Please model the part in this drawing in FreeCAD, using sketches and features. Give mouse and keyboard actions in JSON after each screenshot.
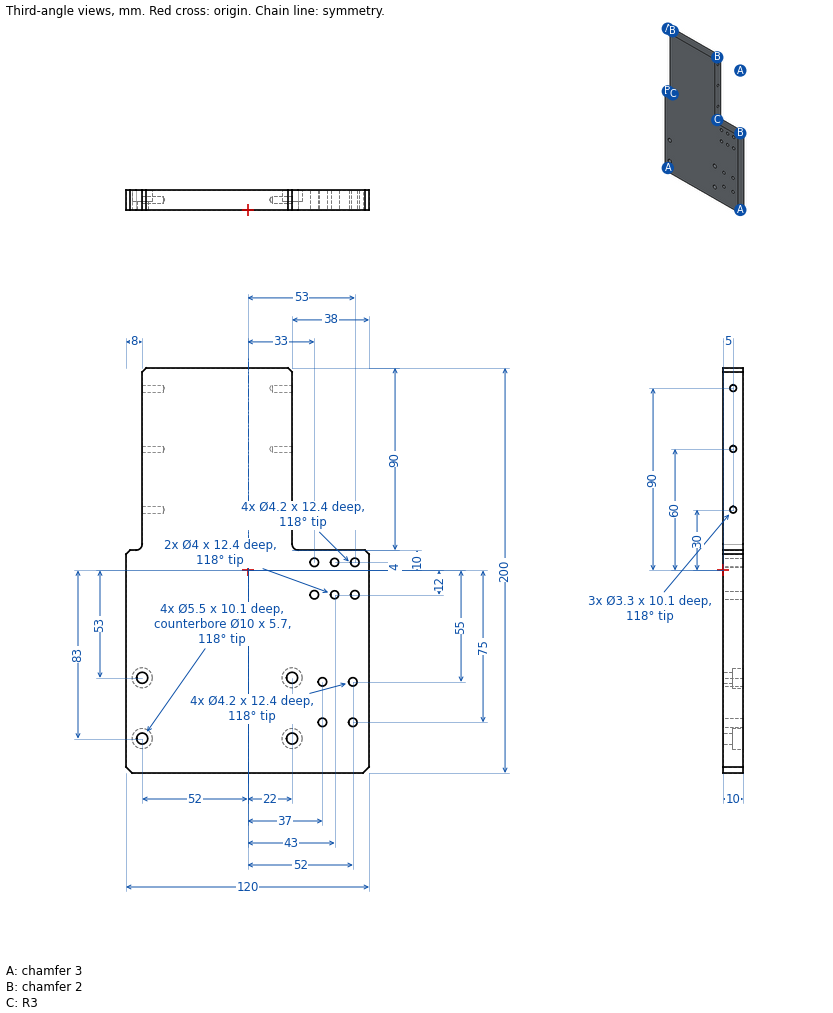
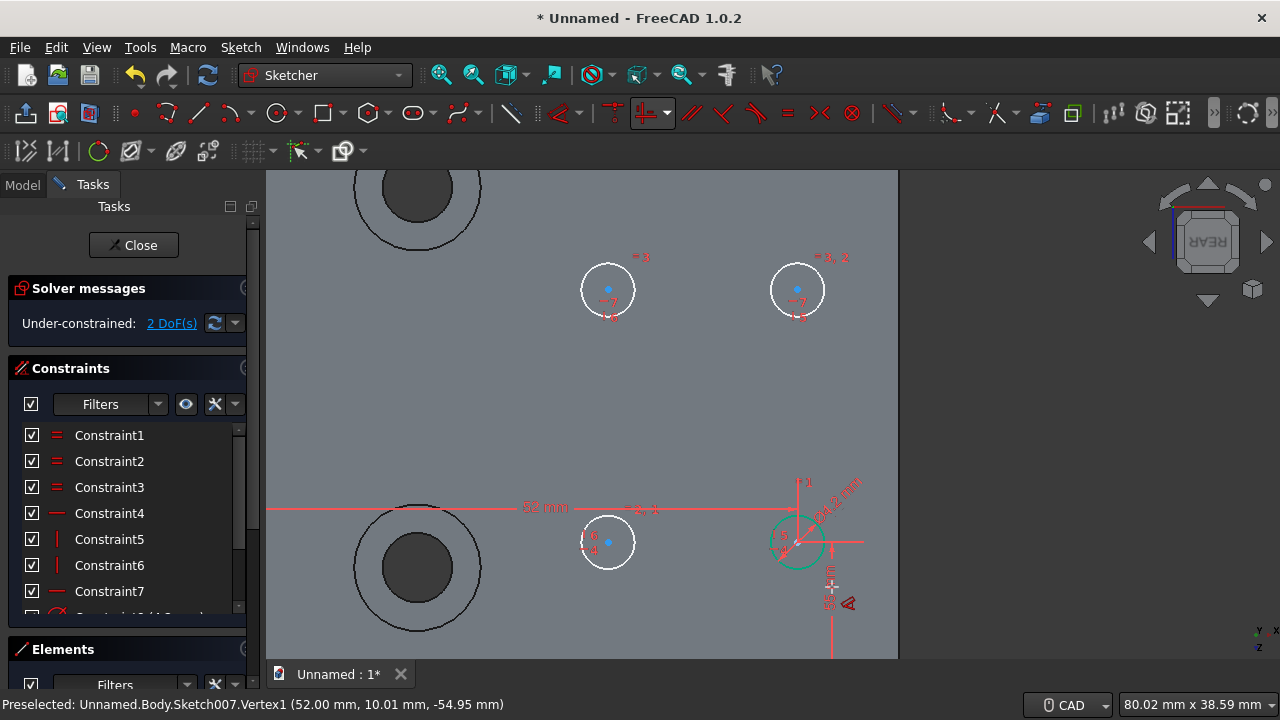
{"action": "left_click", "coordinate": [608, 542]}
{"action": "left_click", "coordinate": [451, 508]}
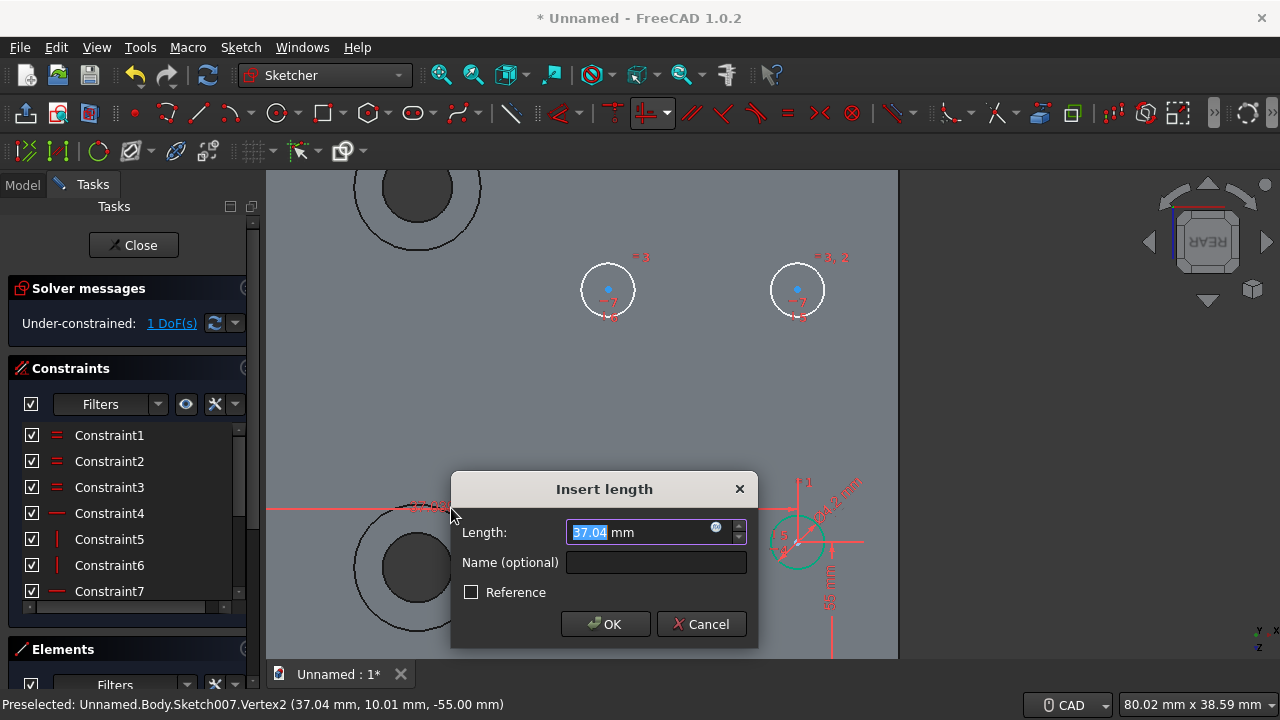
{"action": "type", "text": "37"}
{"action": "key", "text": "Return"}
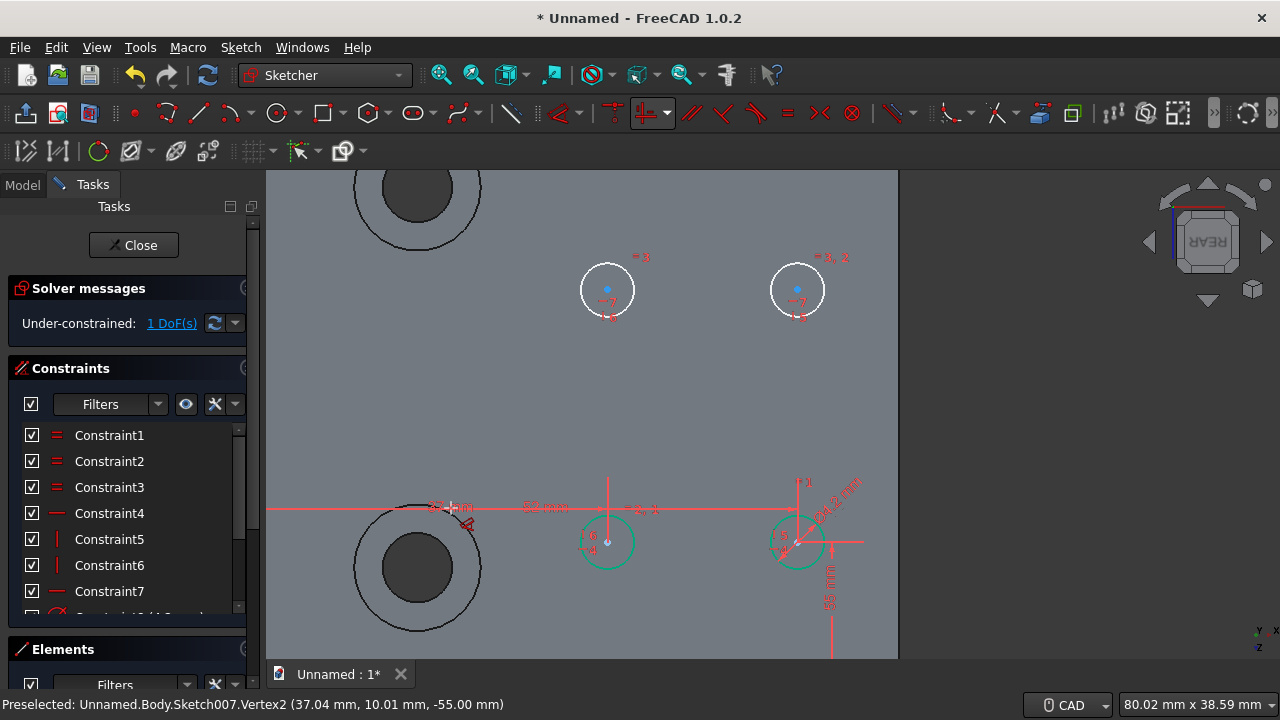
{"action": "left_click", "coordinate": [798, 290]}
{"action": "left_click", "coordinate": [832, 461]}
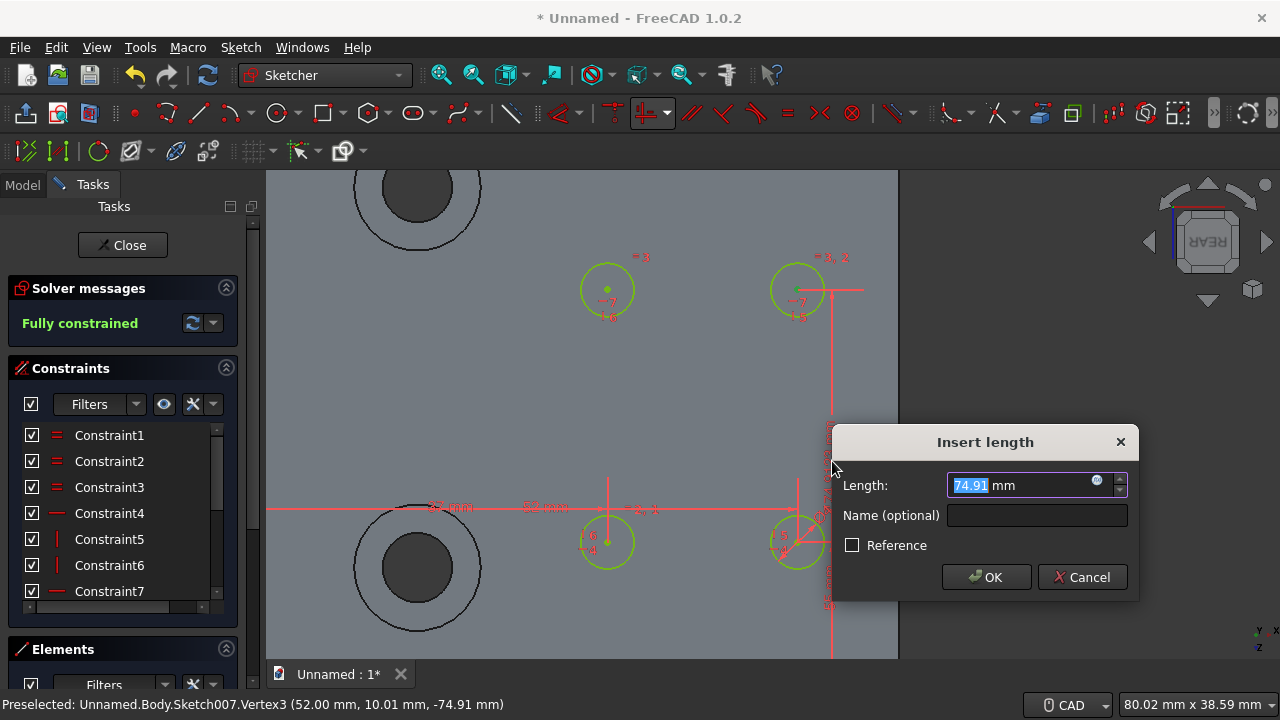
{"action": "type", "text": "75"}
{"action": "key", "text": "Return"}
{"action": "key", "text": "Escape"}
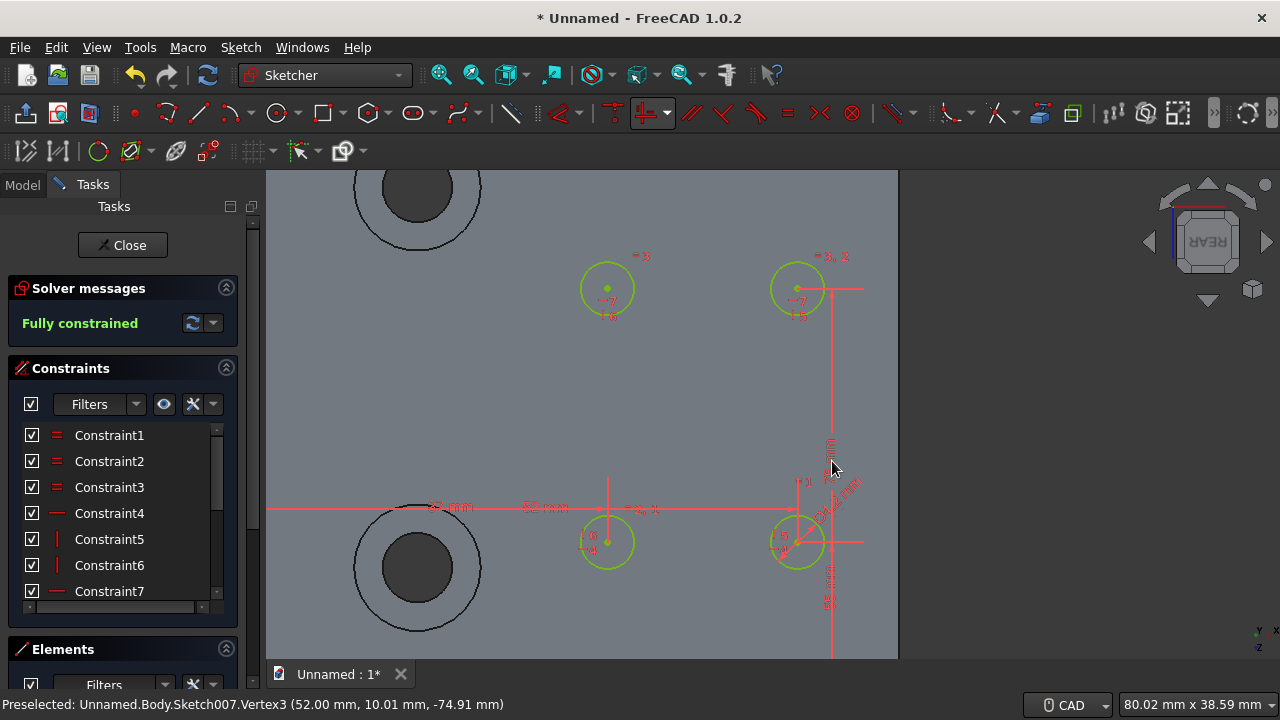
{"action": "left_click", "coordinate": [123, 245]}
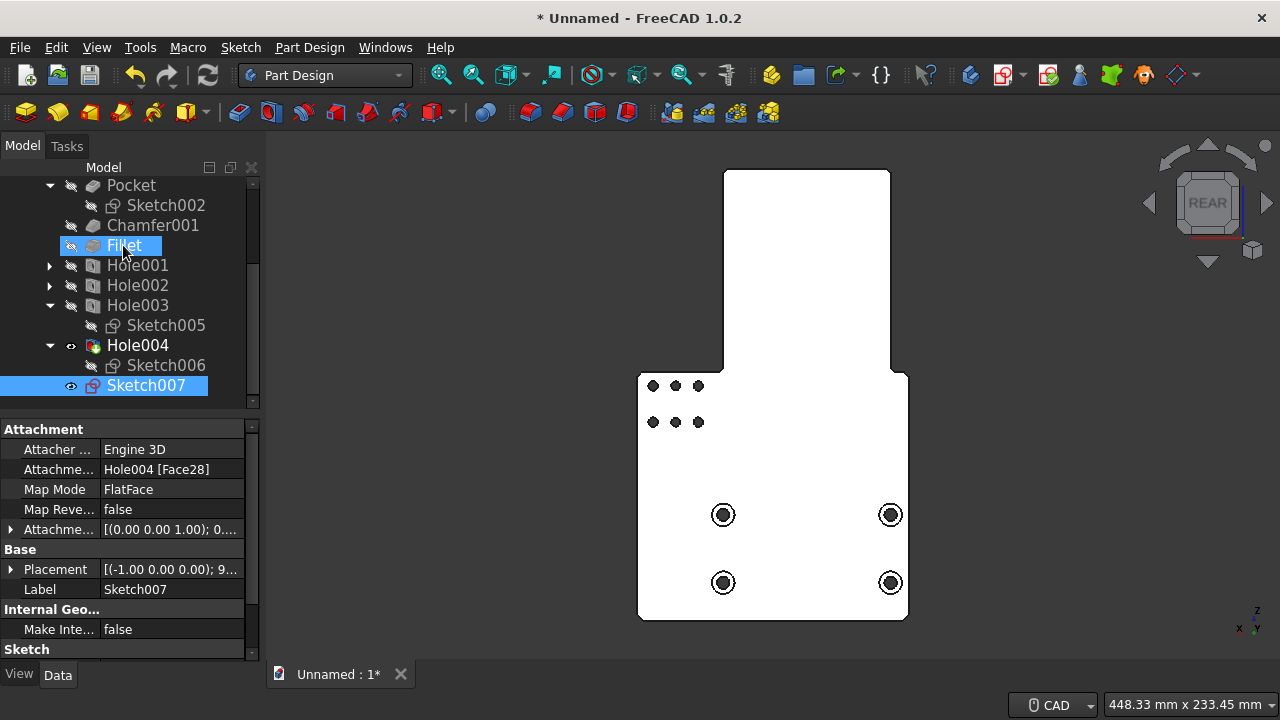
{"action": "left_click", "coordinate": [272, 112]}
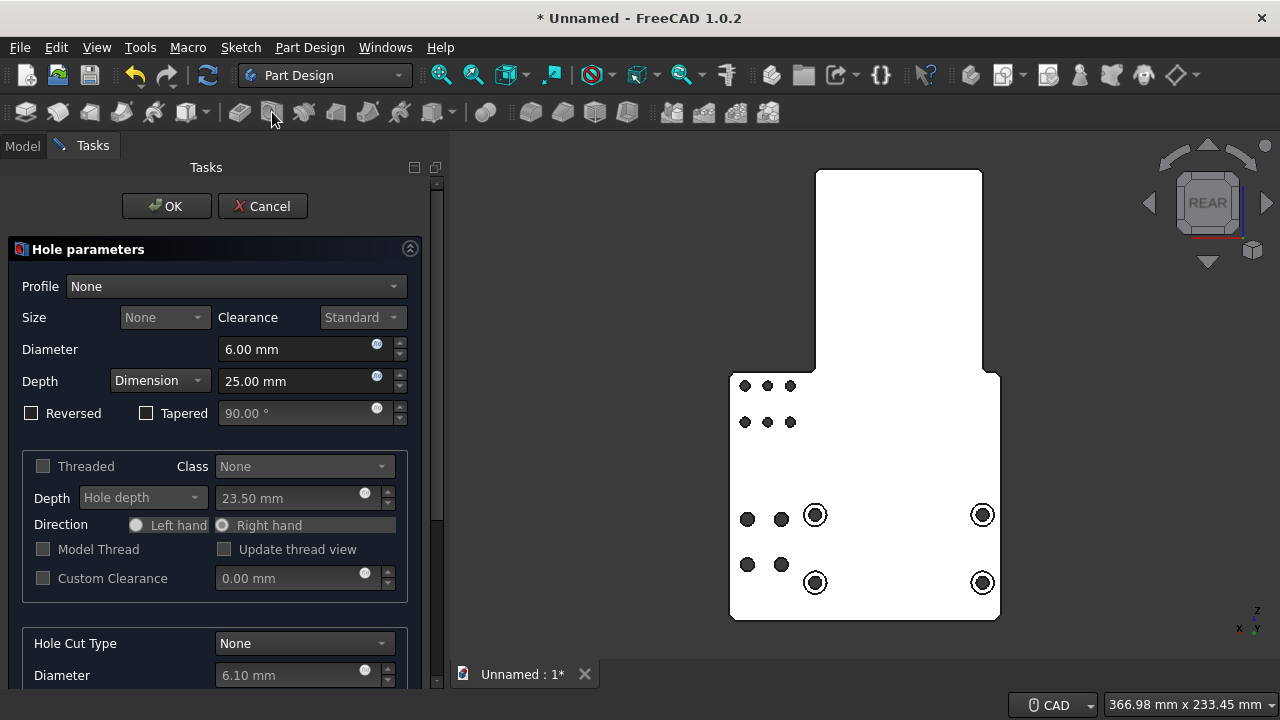
{"action": "triple_click", "coordinate": [305, 349]}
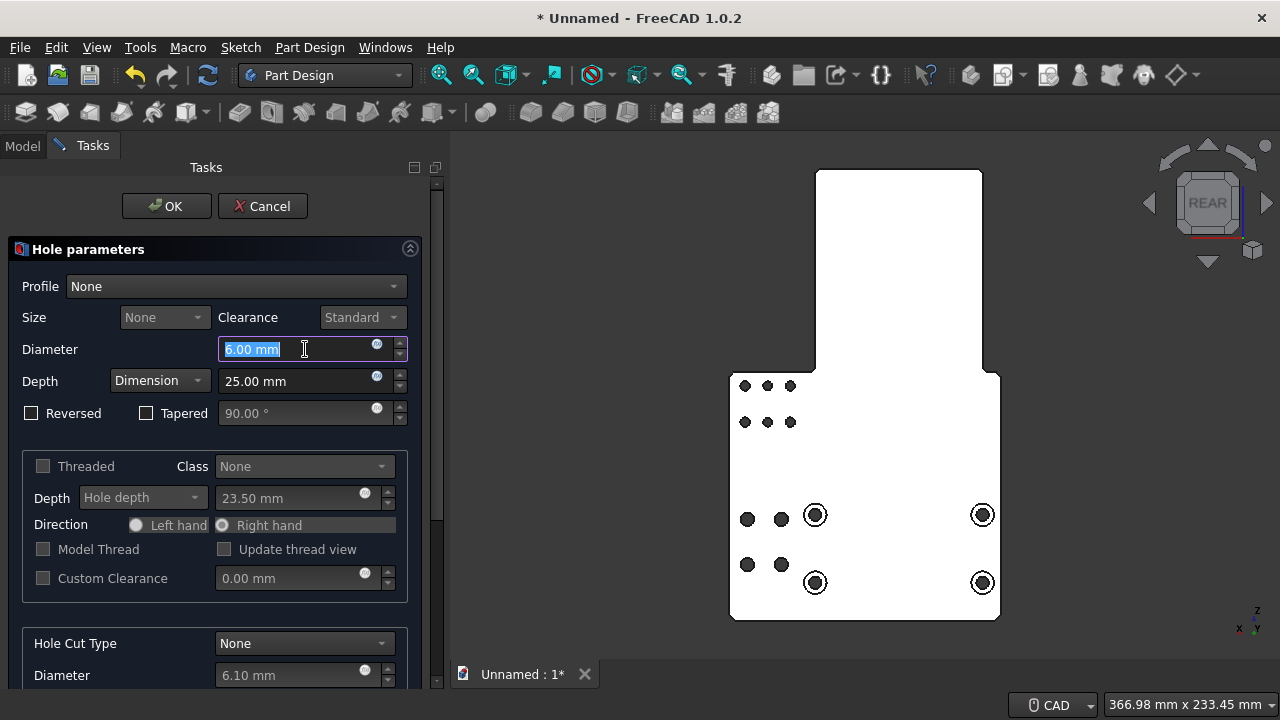
{"action": "type", "text": "4.2"}
{"action": "key", "text": "Tab"}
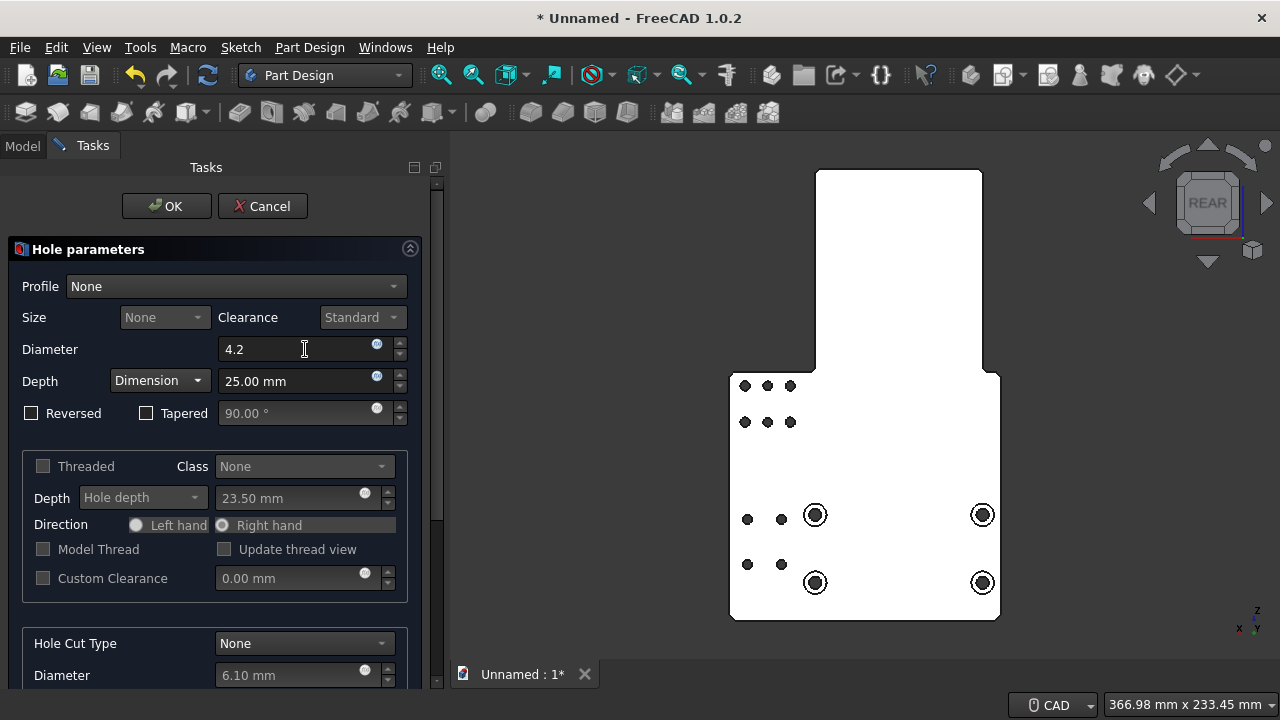
{"action": "triple_click", "coordinate": [305, 381]}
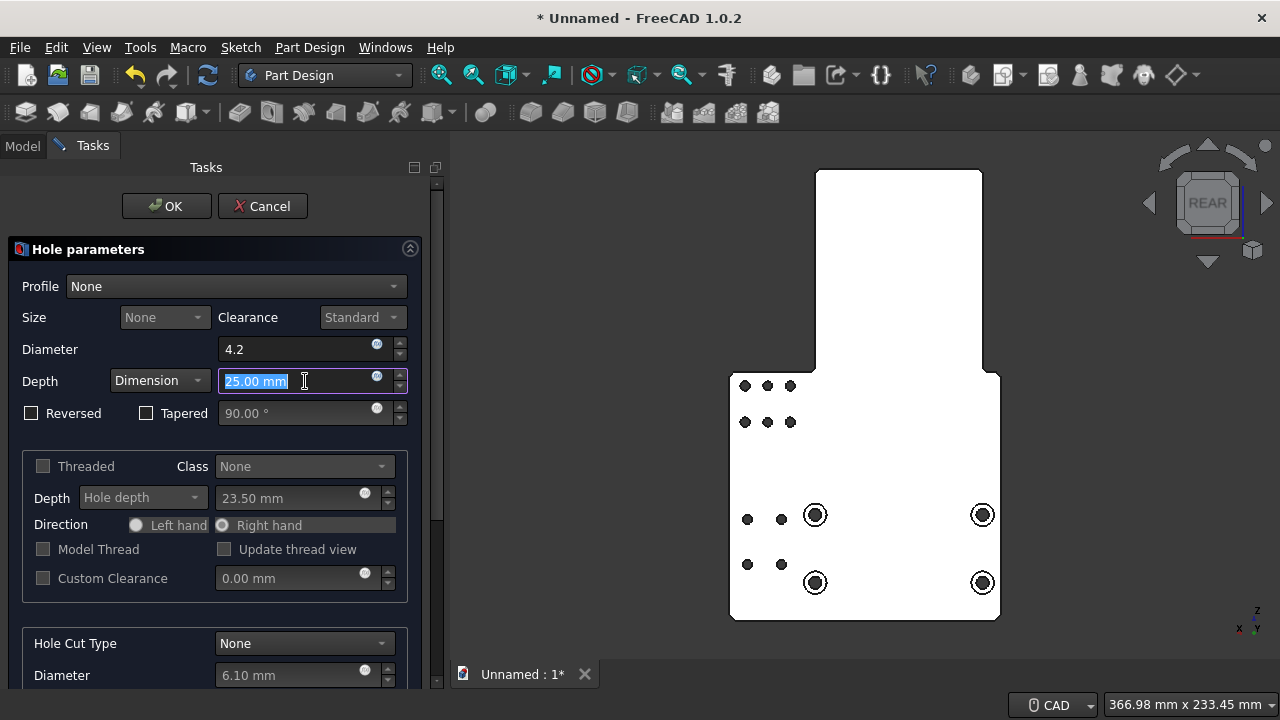
{"action": "type", "text": "12.4"}
{"action": "key", "text": "Tab"}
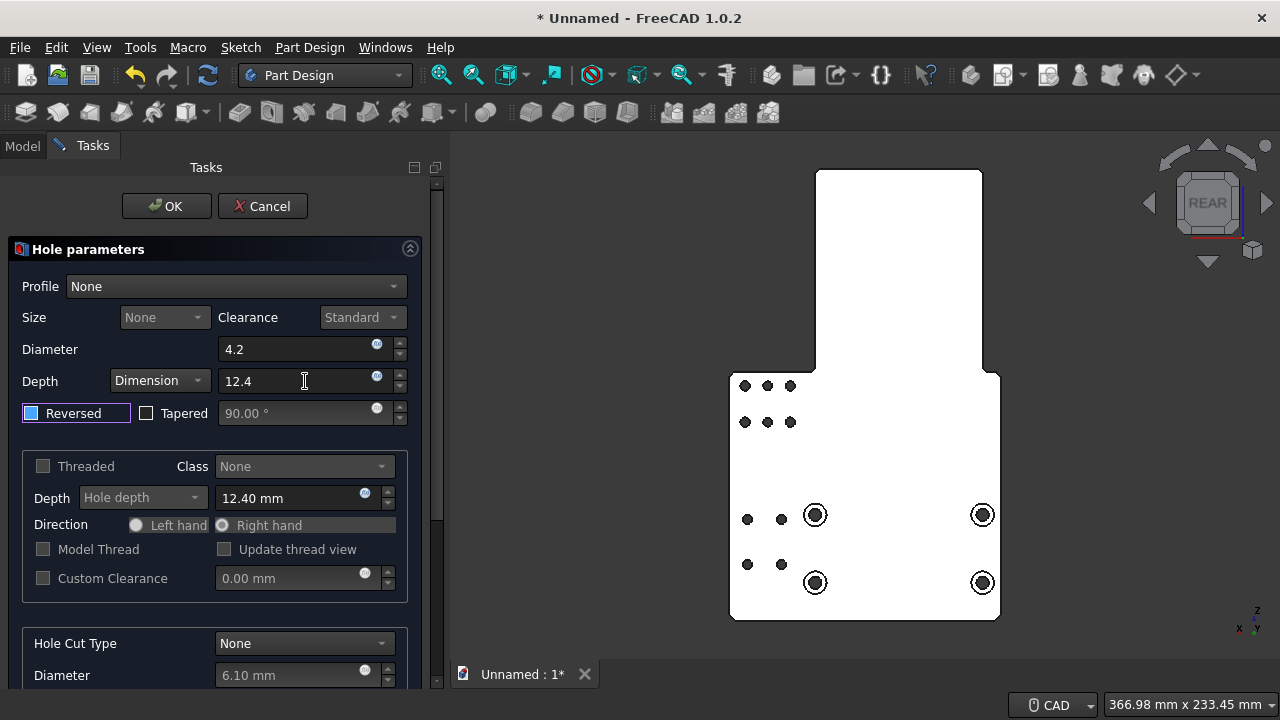
{"action": "left_click", "coordinate": [167, 206]}